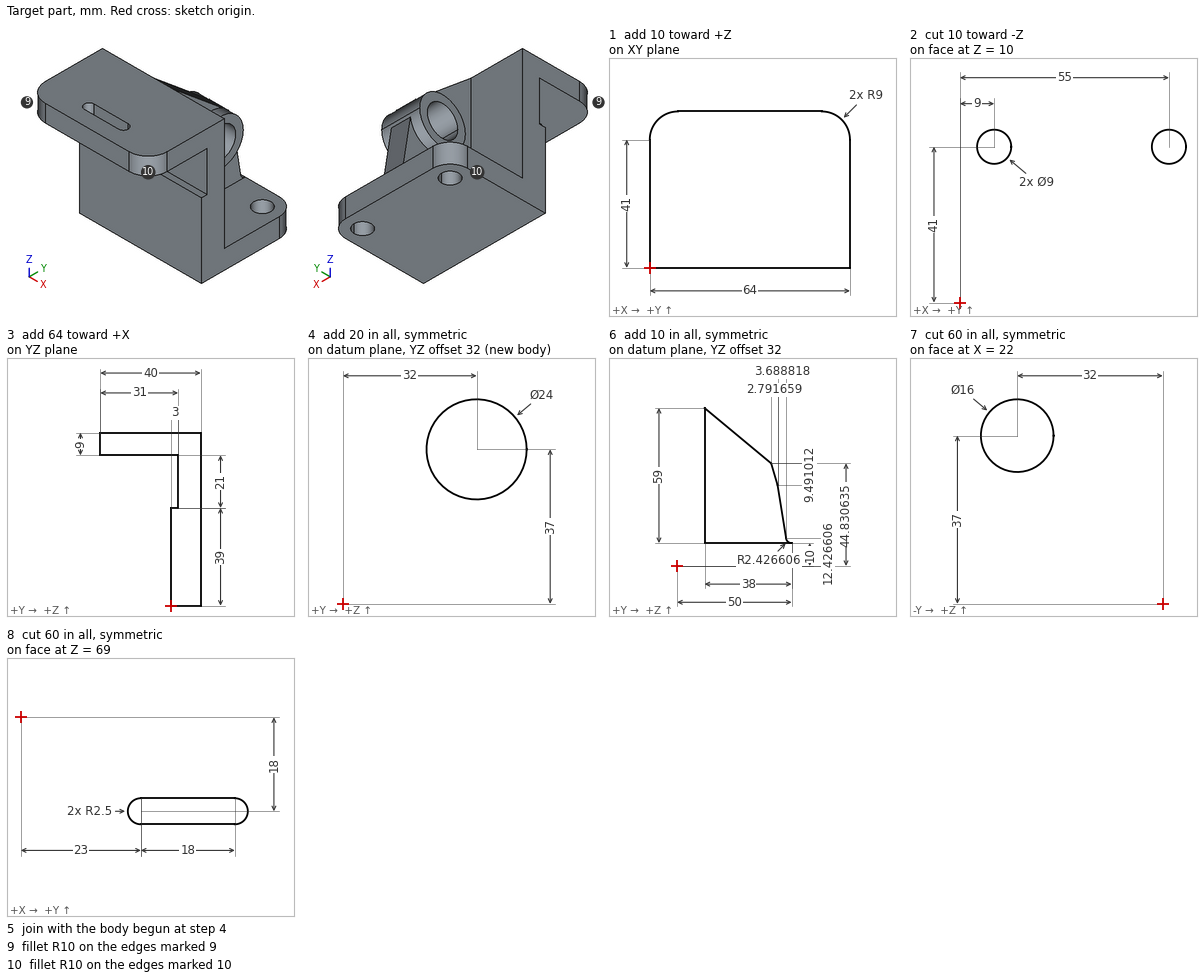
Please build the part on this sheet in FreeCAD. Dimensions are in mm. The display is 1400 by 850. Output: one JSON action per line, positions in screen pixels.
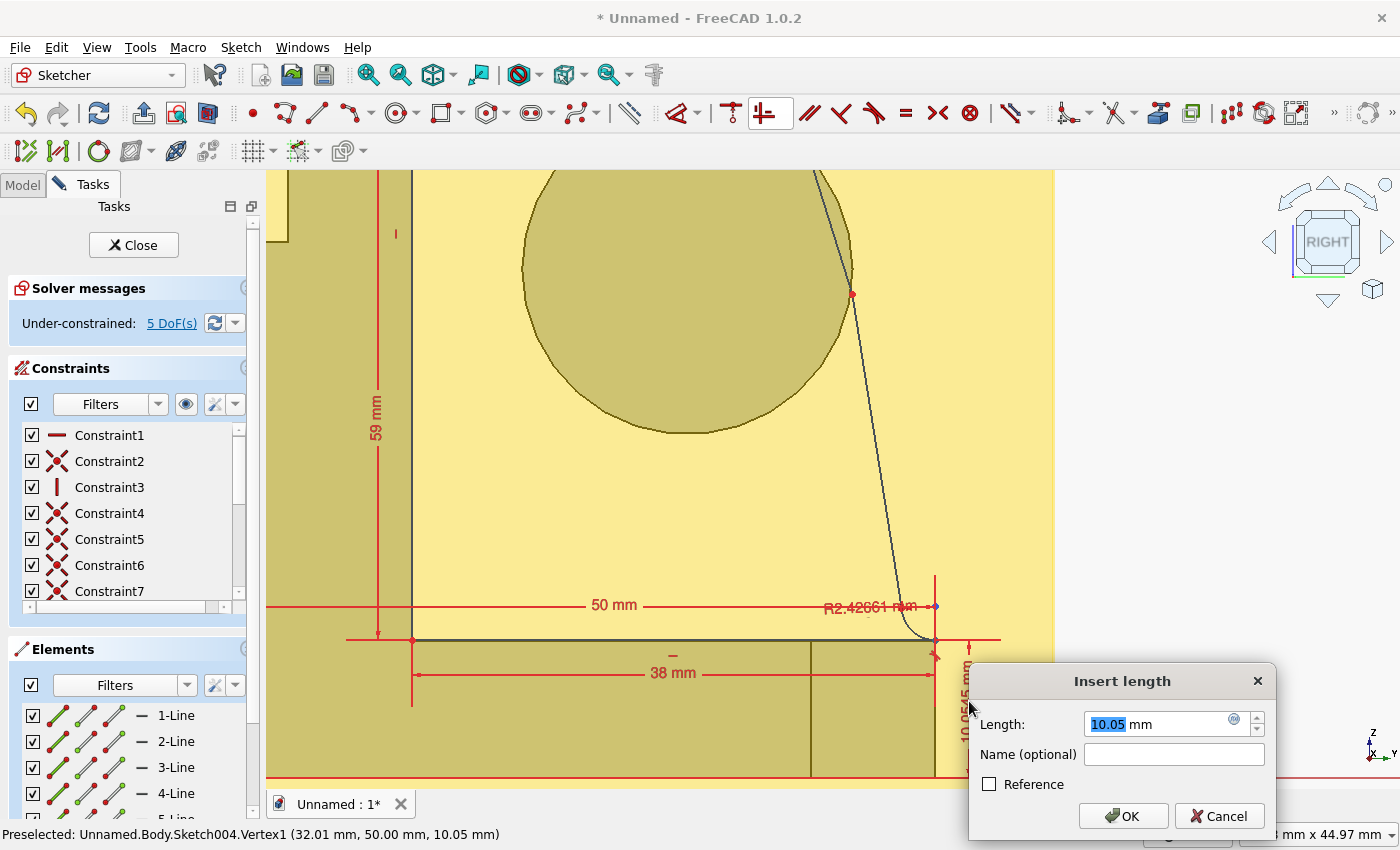
{"action": "type", "text": "10"}
{"action": "key", "text": "Return"}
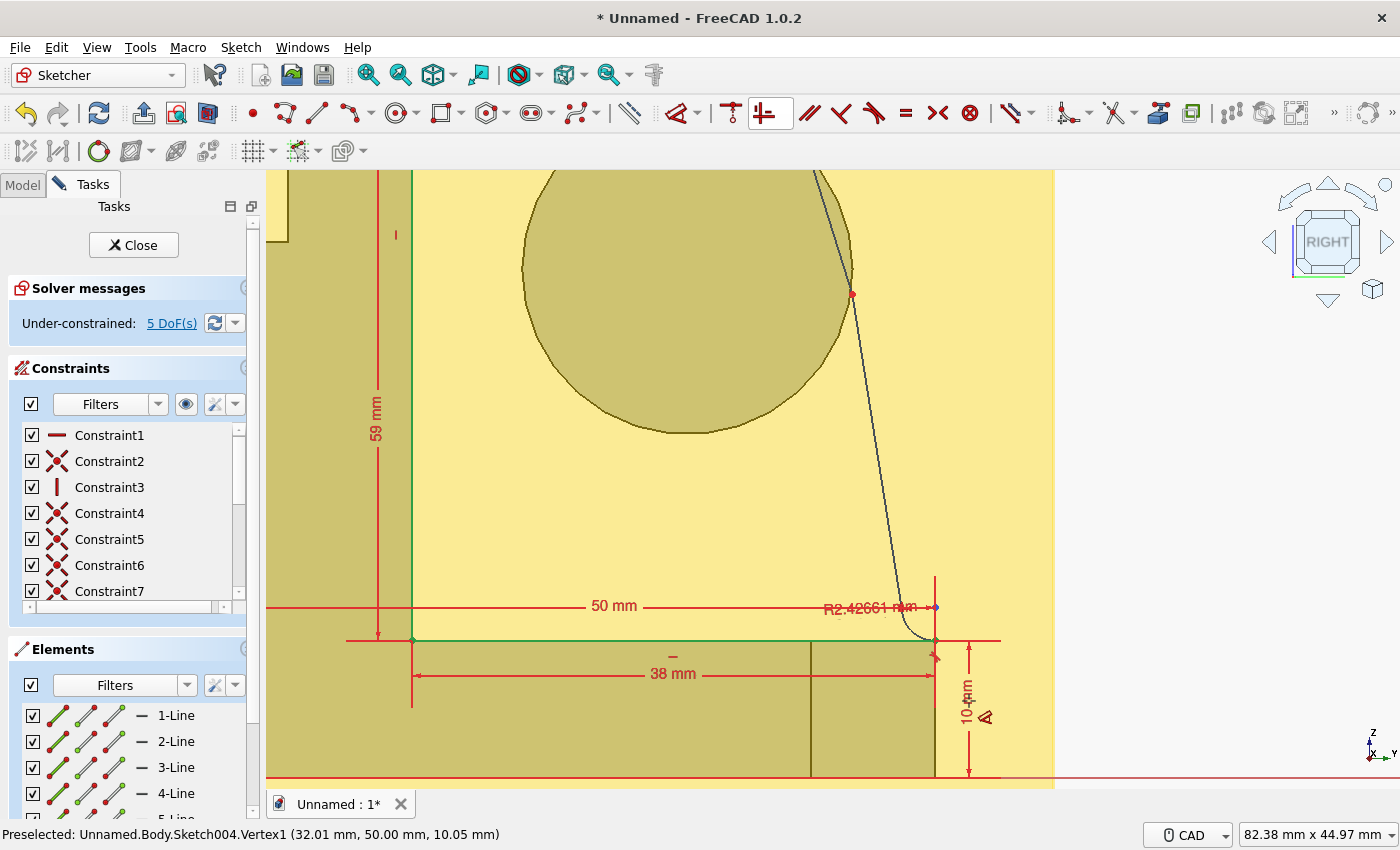
{"action": "left_click", "coordinate": [824, 203]}
{"action": "left_click", "coordinate": [832, 328]}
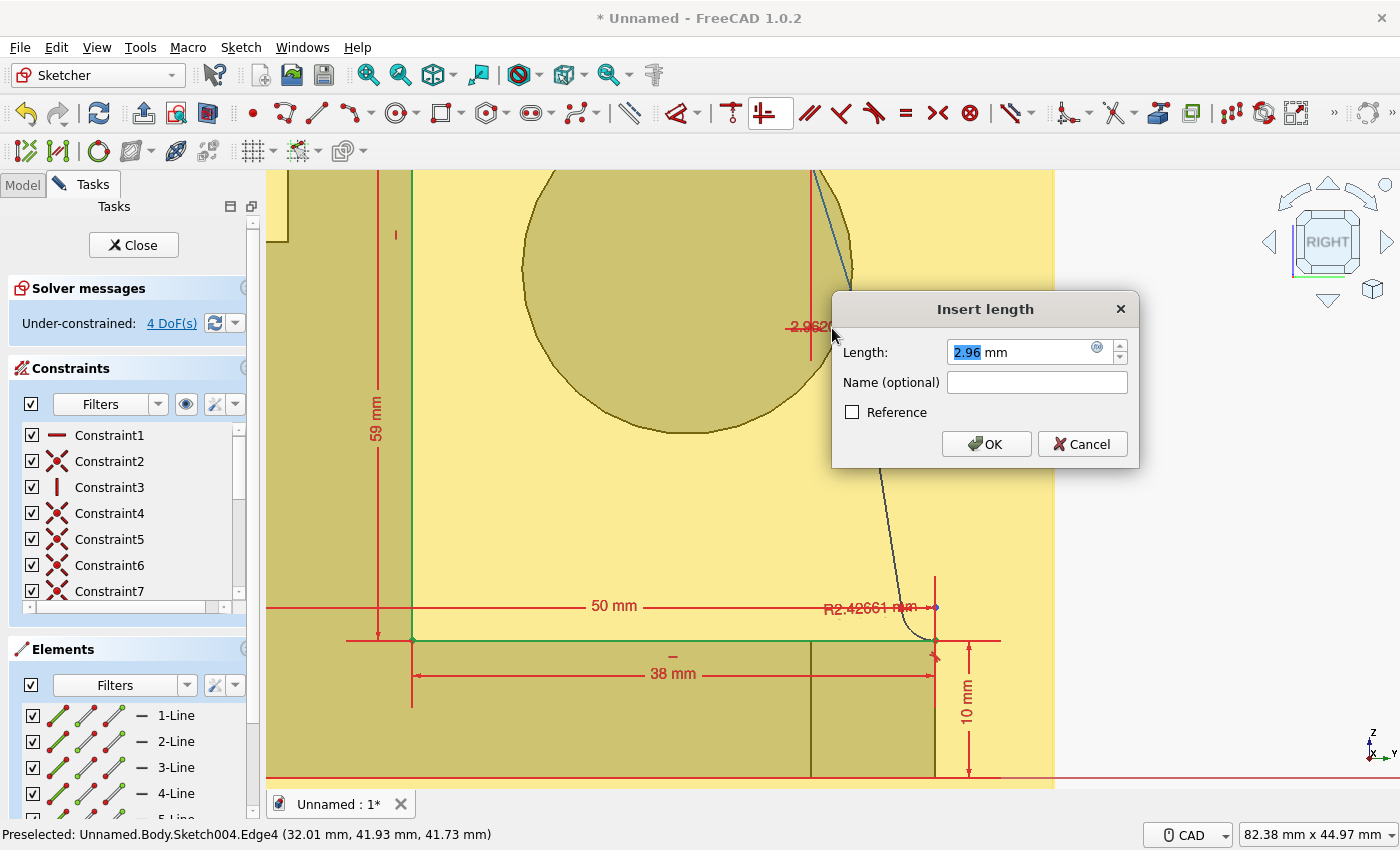
{"action": "type", "text": "2.791659"}
{"action": "key", "text": "Return"}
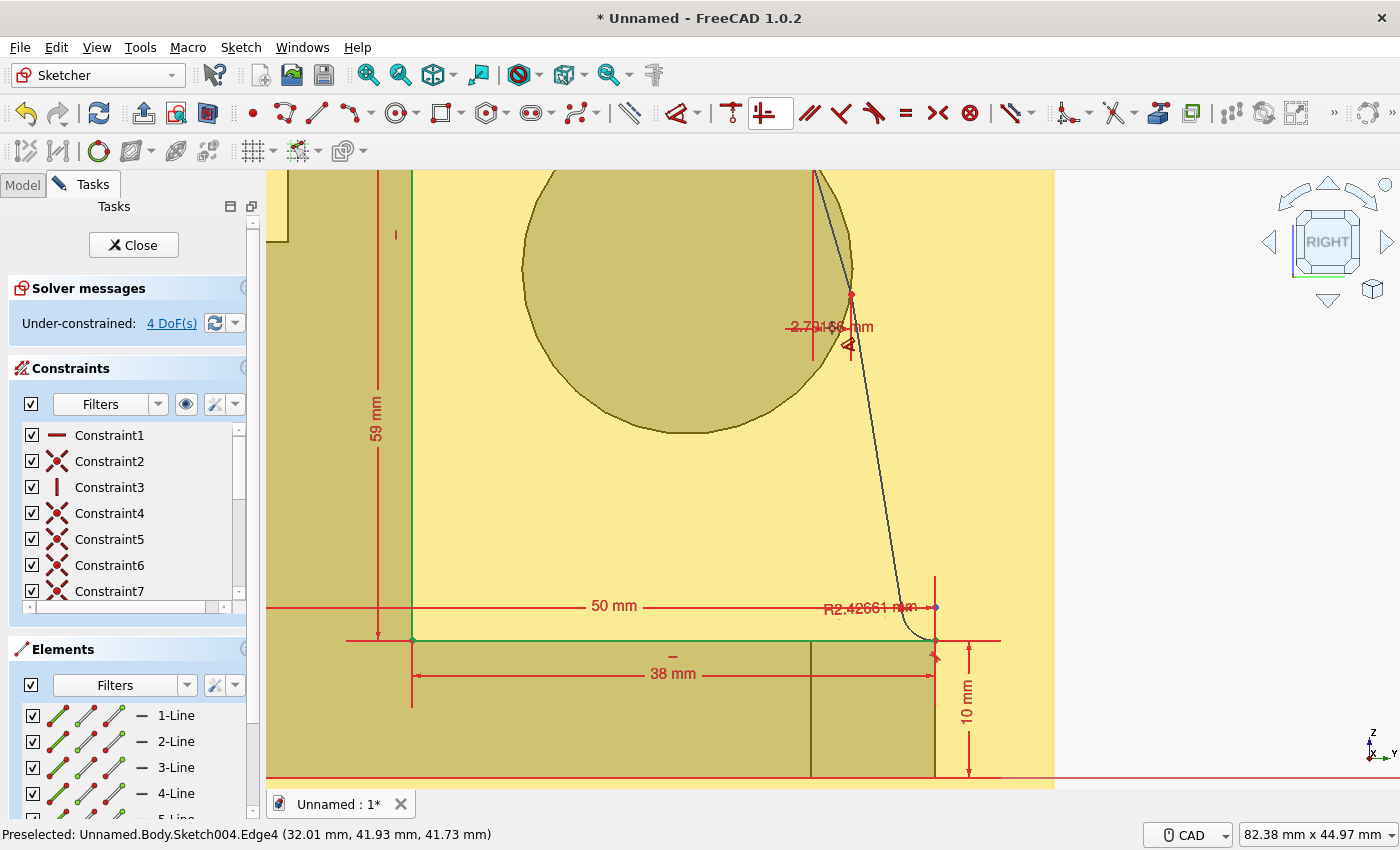
{"action": "left_click", "coordinate": [824, 203]}
{"action": "left_click", "coordinate": [885, 246]}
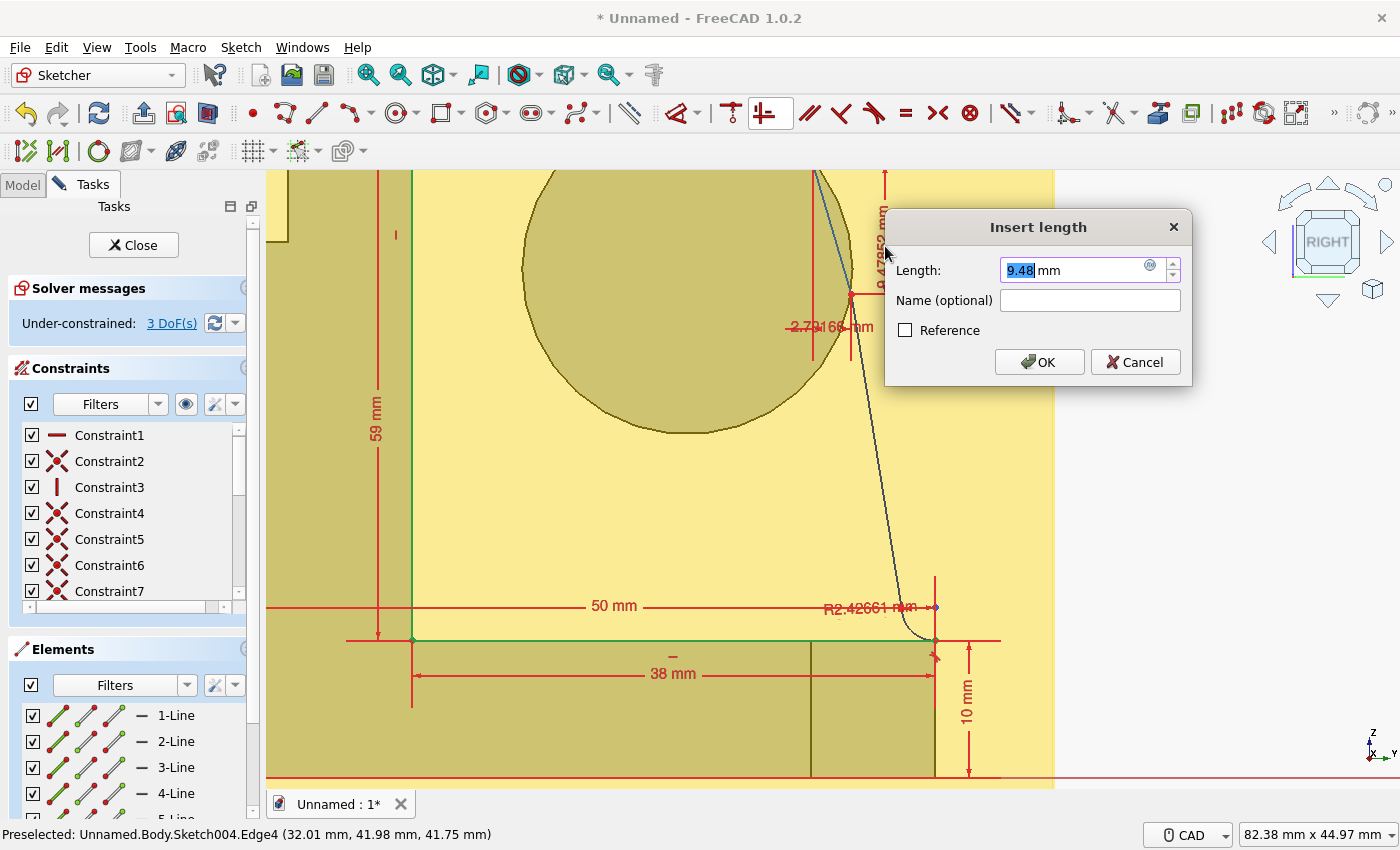
{"action": "type", "text": "9.491012"}
{"action": "key", "text": "Return"}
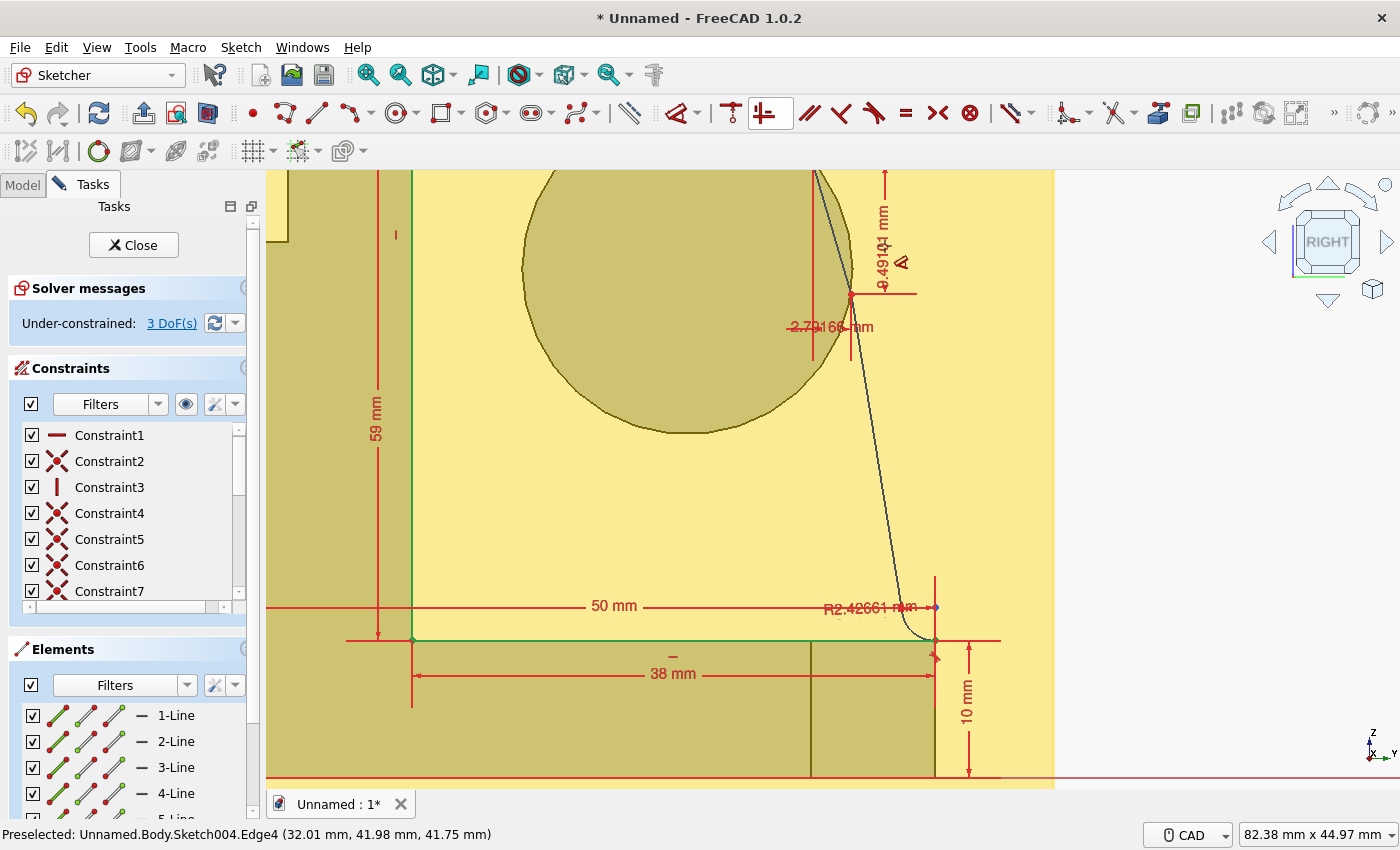
{"action": "left_click", "coordinate": [866, 389]}
{"action": "left_click", "coordinate": [877, 667]}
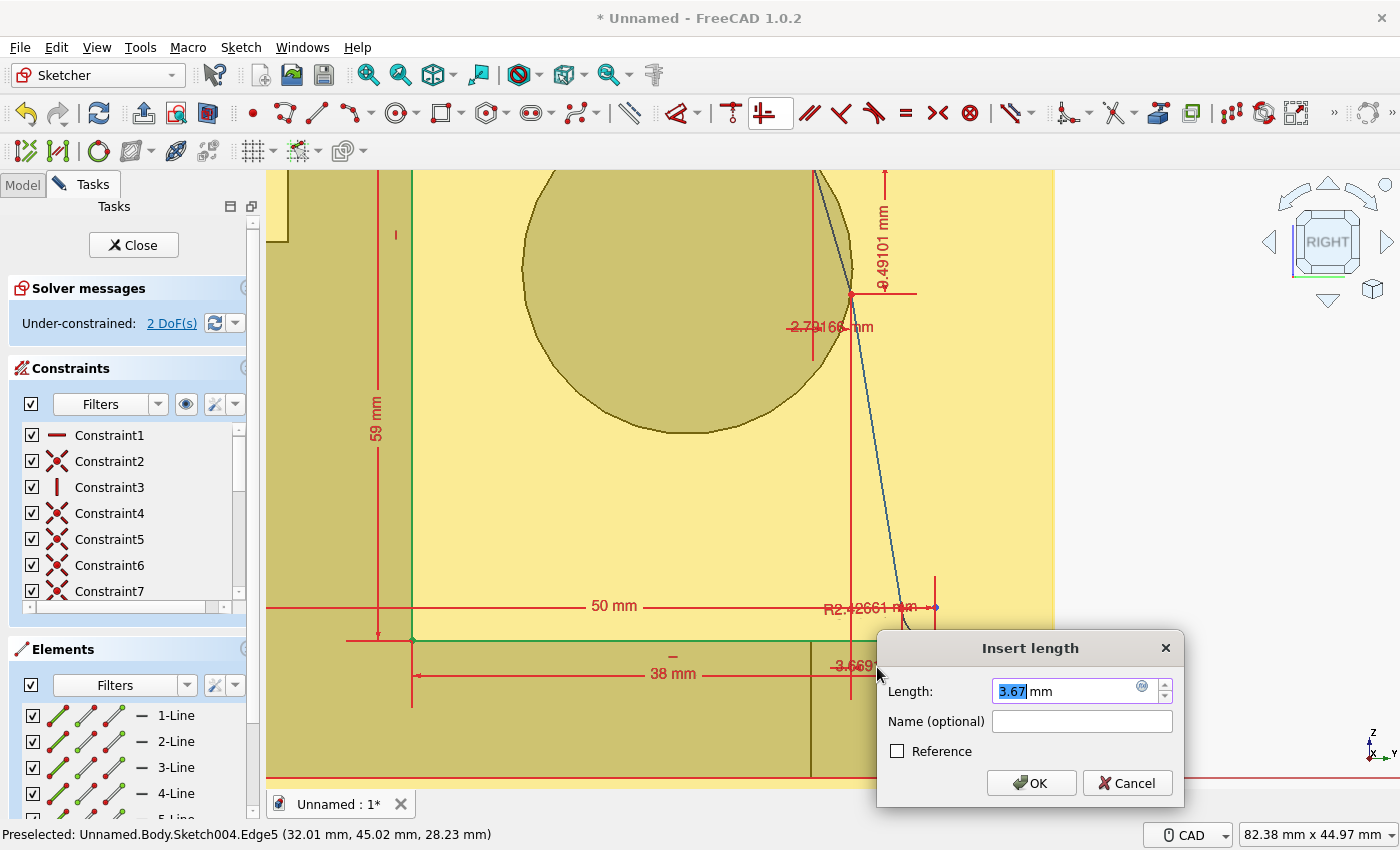
{"action": "type", "text": "3.688818"}
{"action": "key", "text": "Return"}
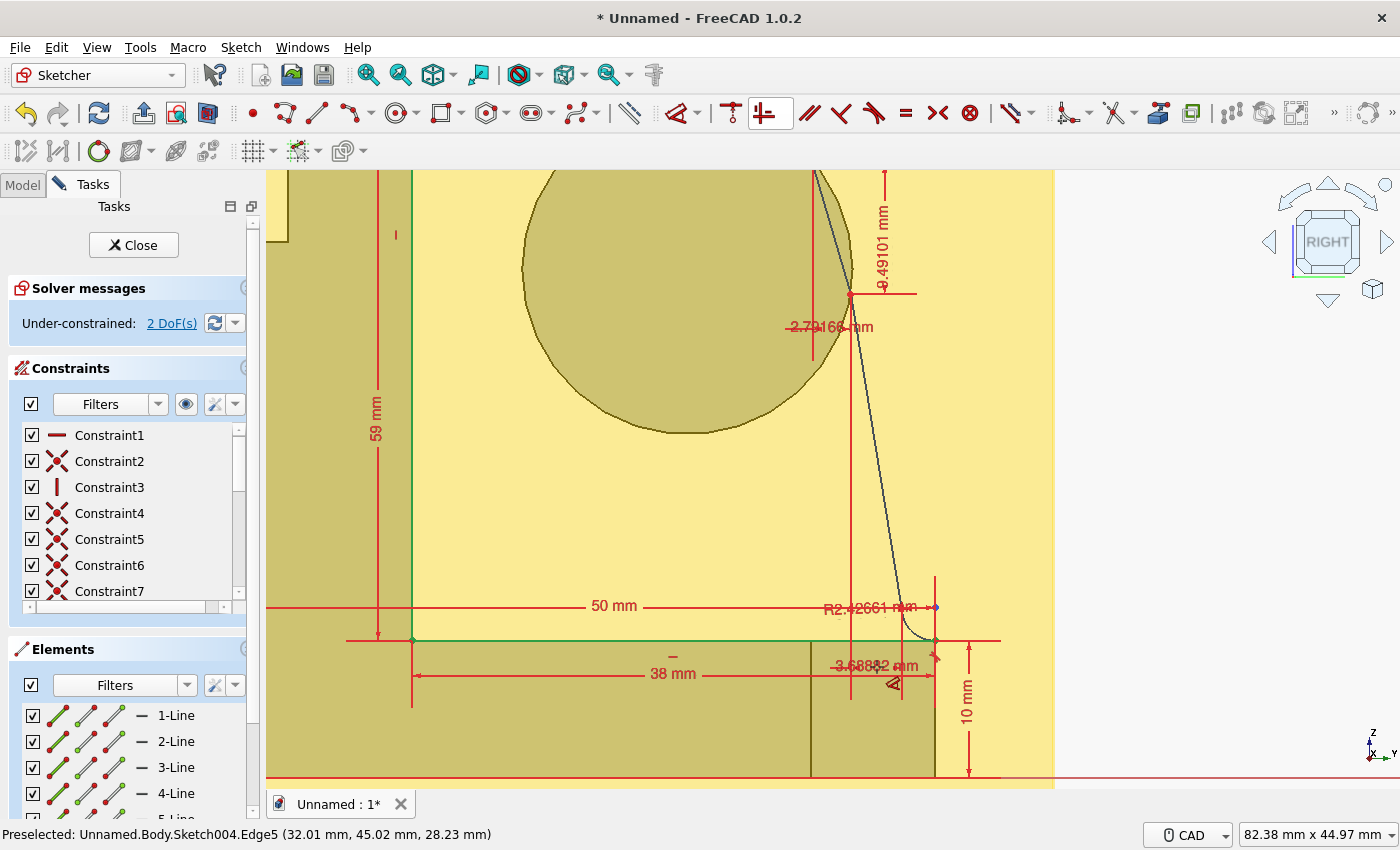
{"action": "scroll", "coordinate": [906, 623], "scroll_direction": "down", "scroll_amount": 4}